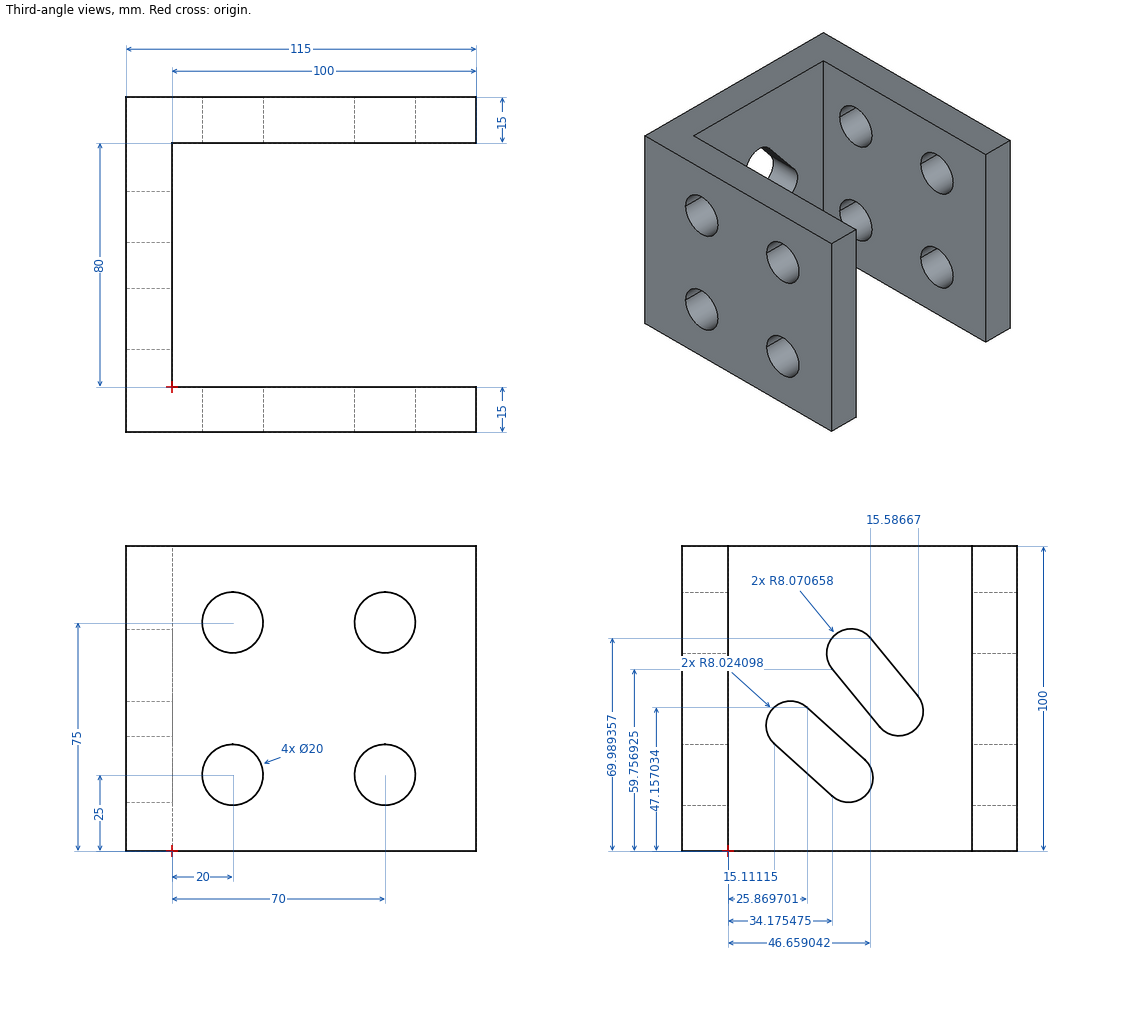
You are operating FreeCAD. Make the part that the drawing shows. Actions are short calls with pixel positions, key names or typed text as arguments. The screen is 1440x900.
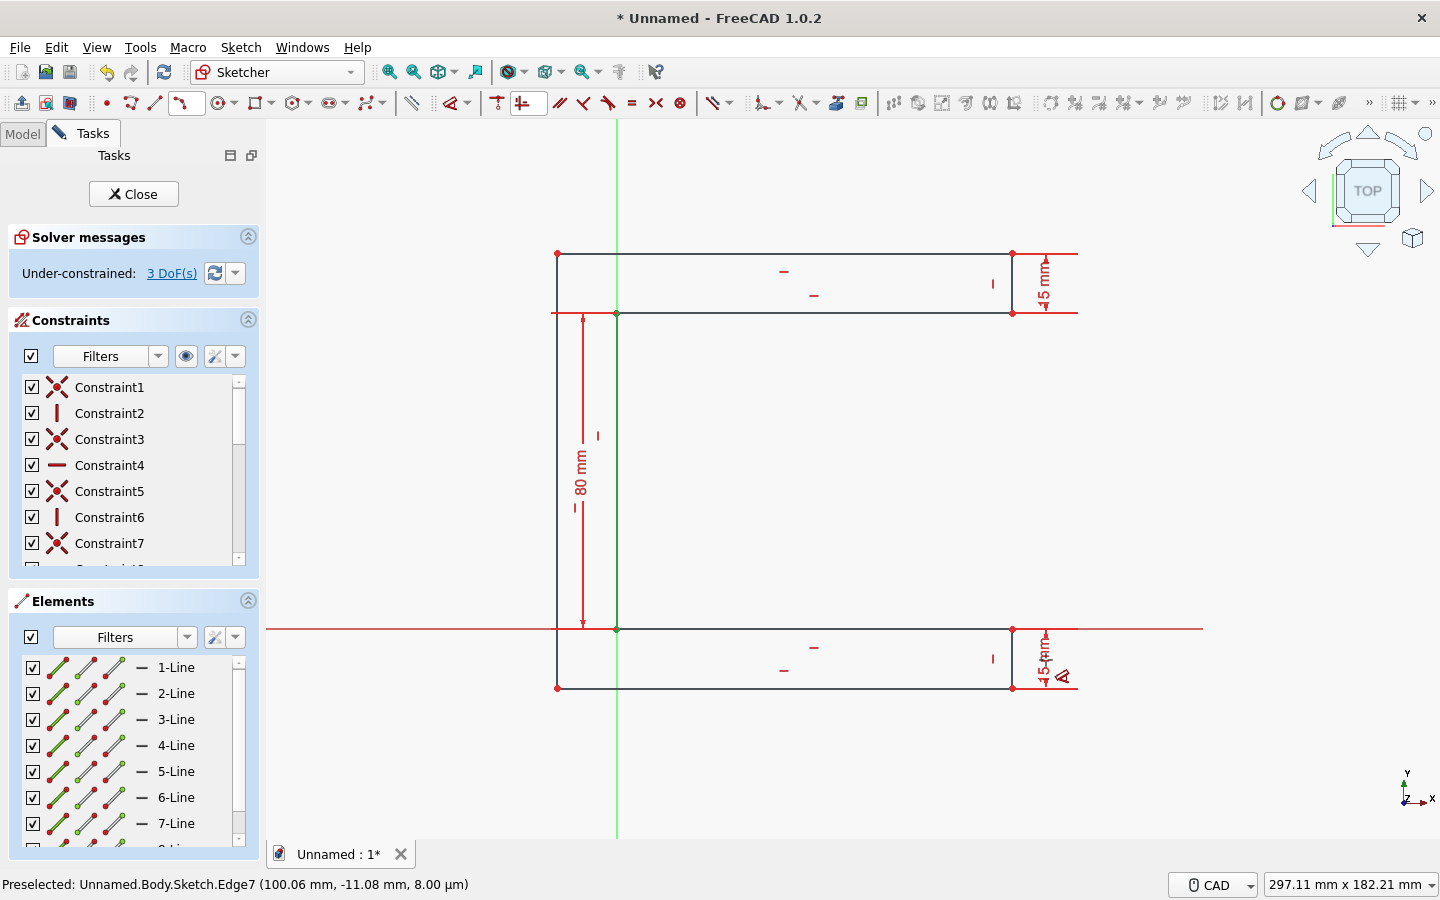
click(735, 313)
click(814, 279)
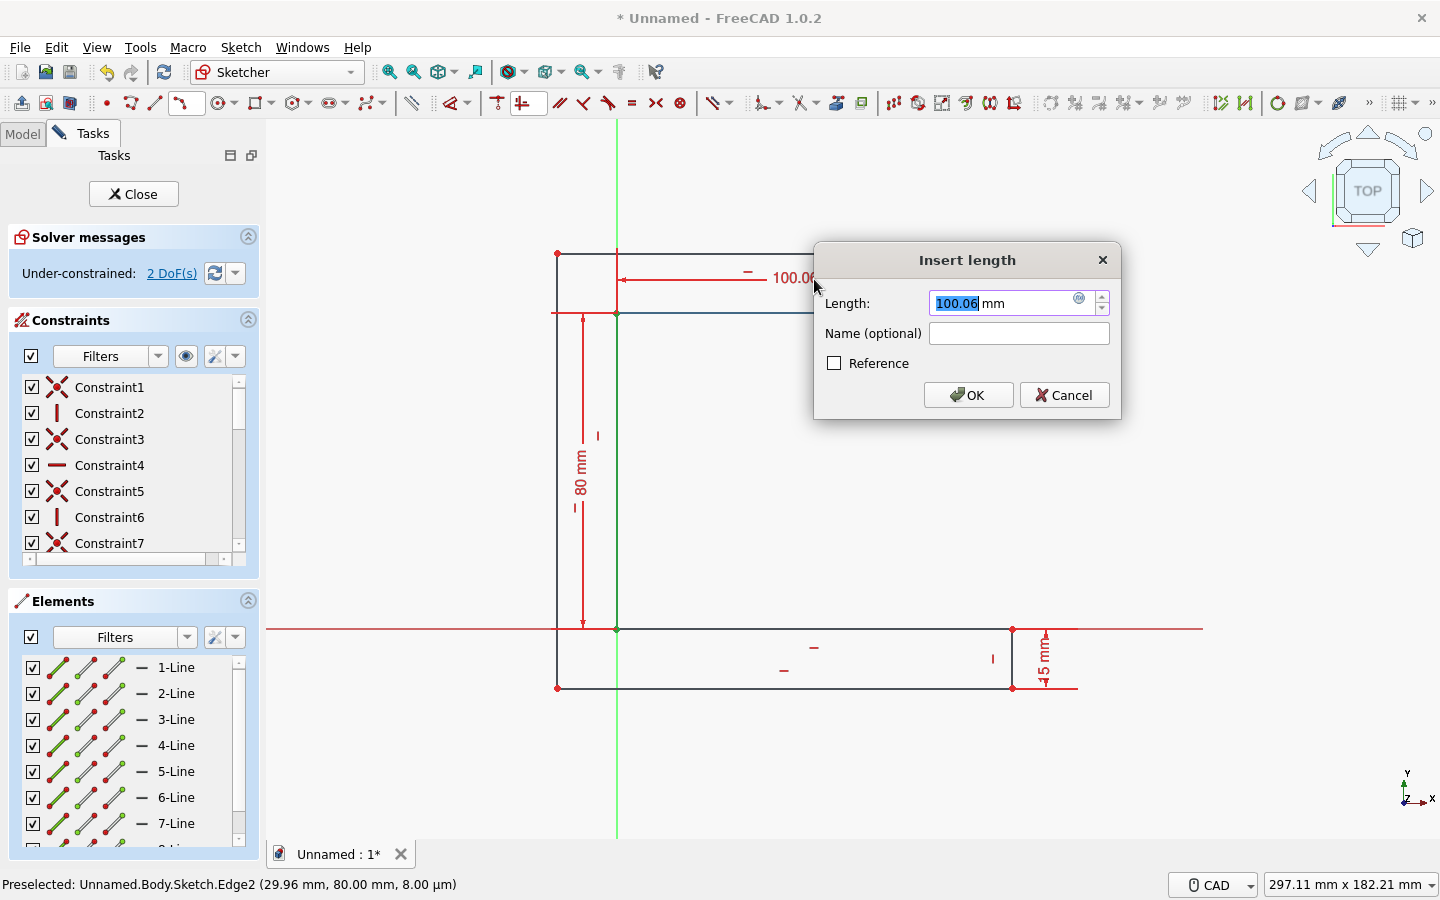
text(100)
key(Return)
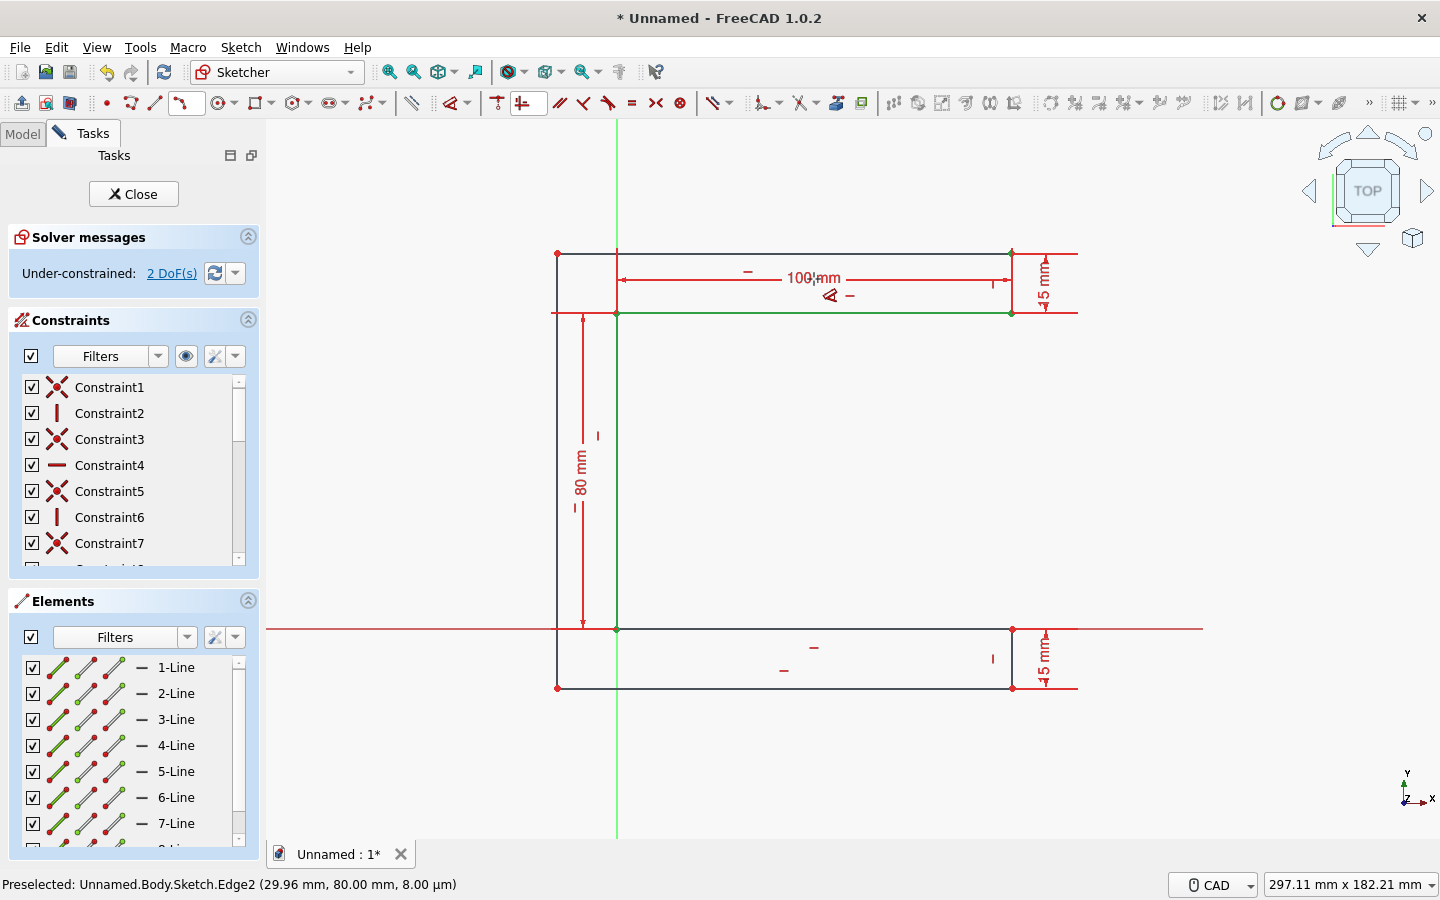
click(875, 254)
click(784, 220)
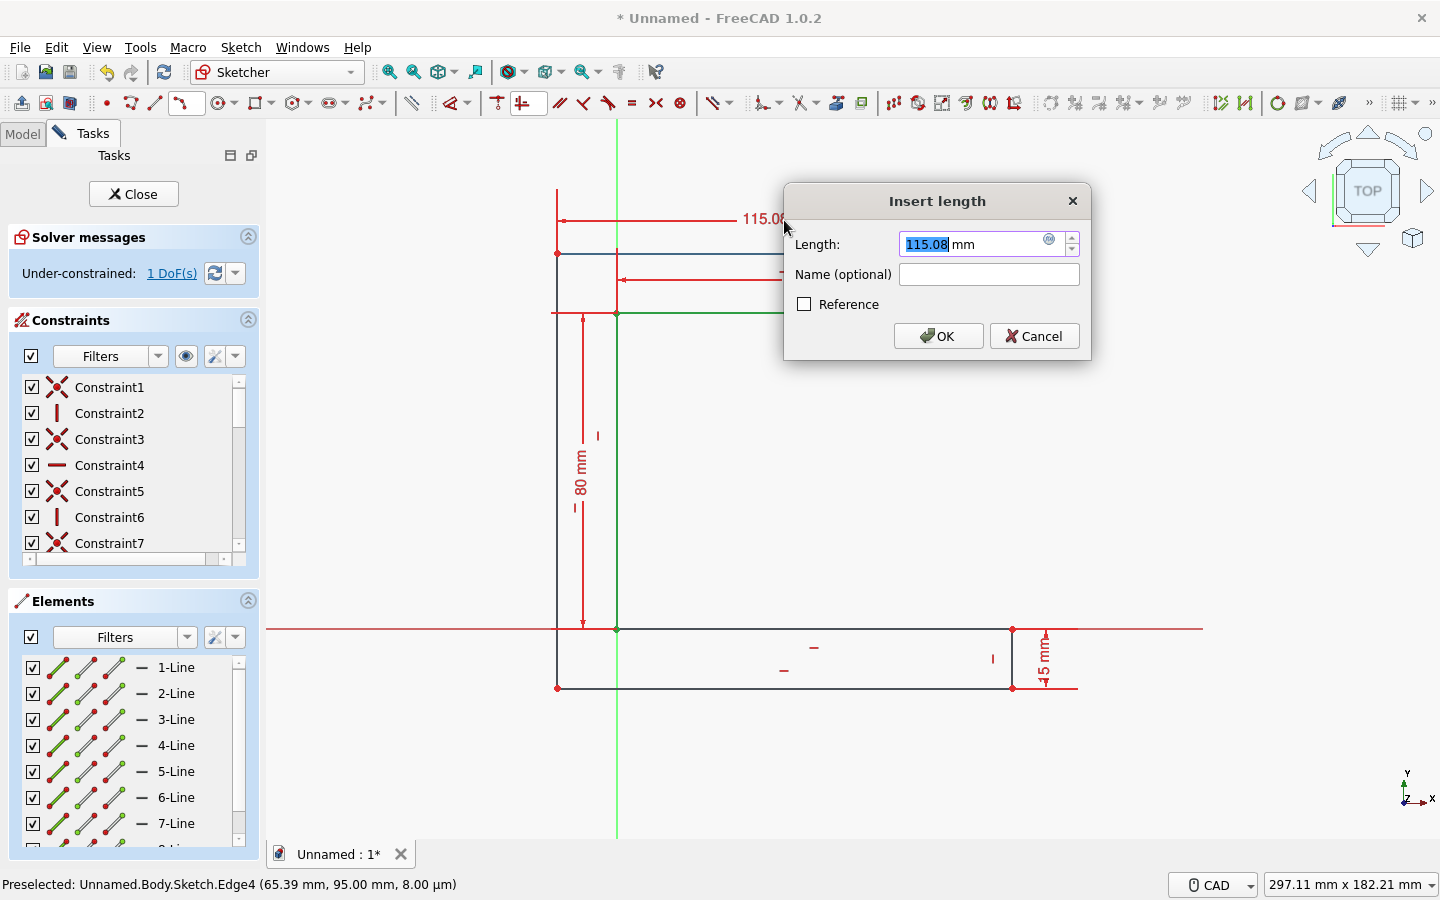
text(115)
key(Return)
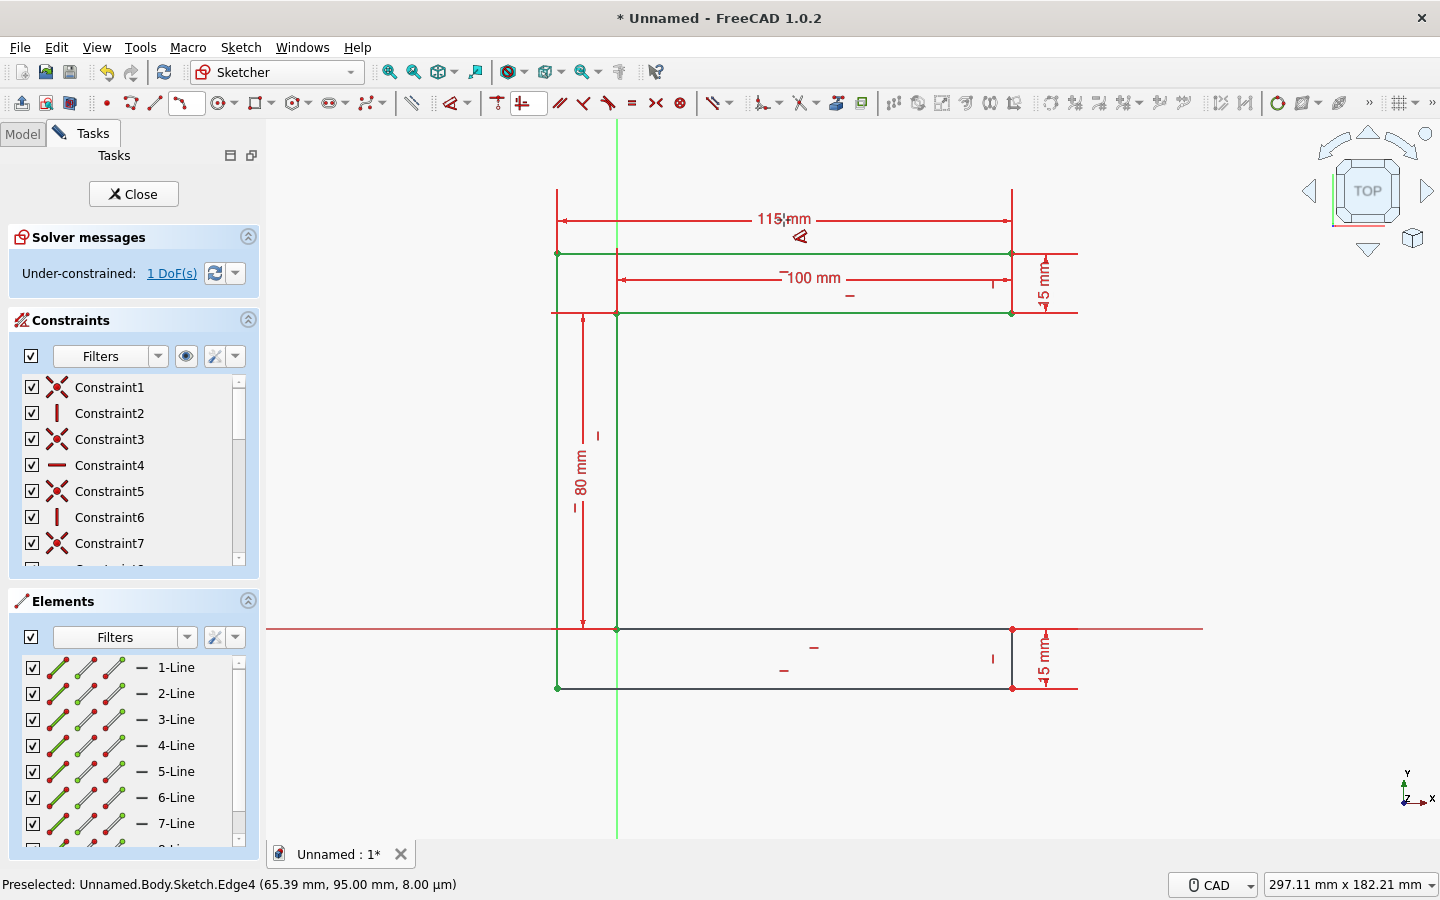
click(694, 689)
click(785, 723)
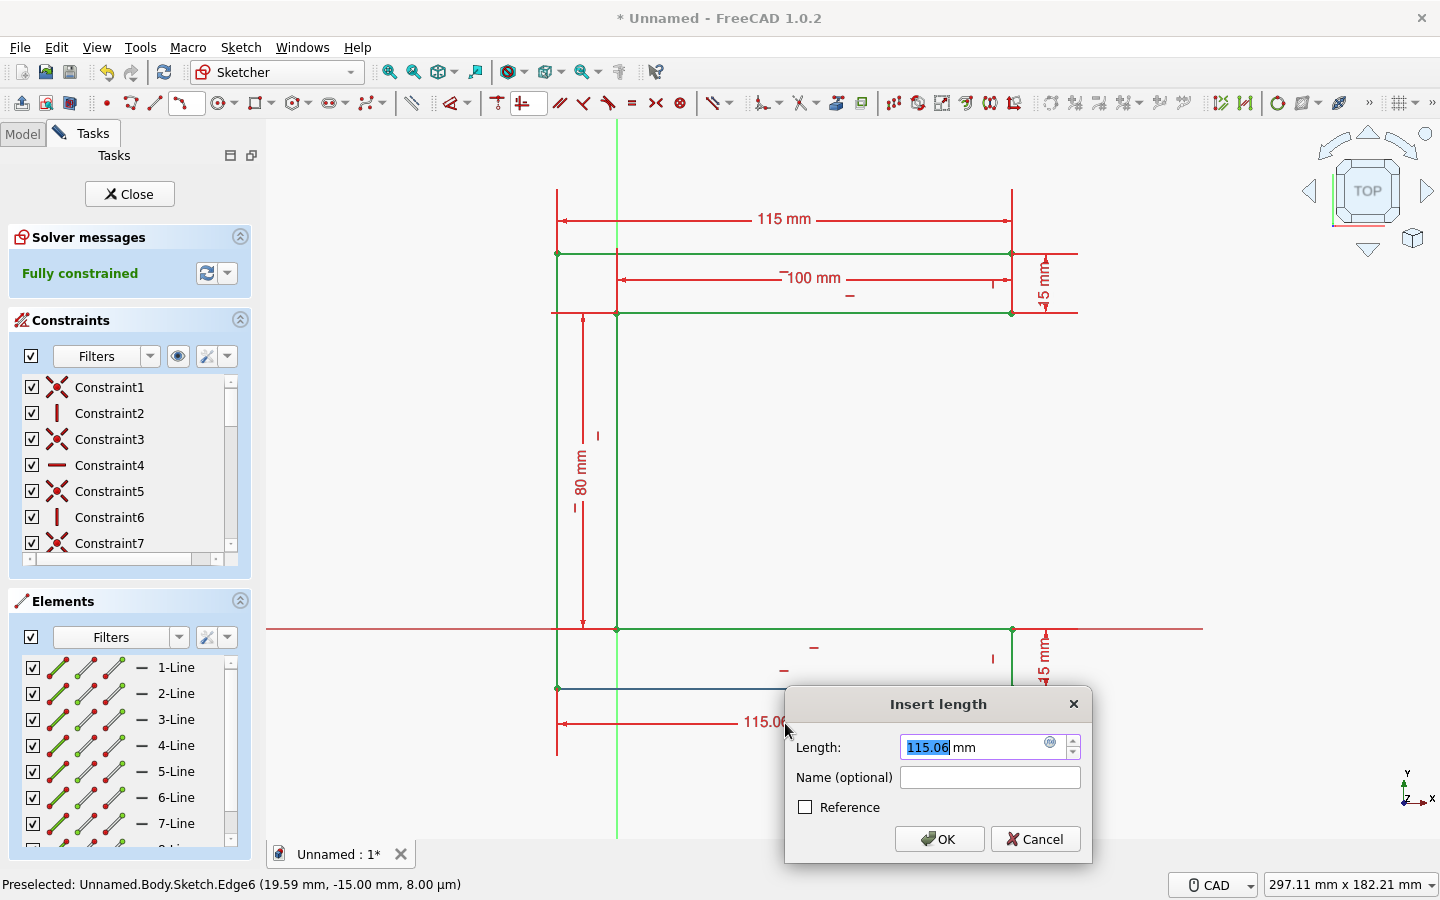
text(115)
key(Return)
key(Escape)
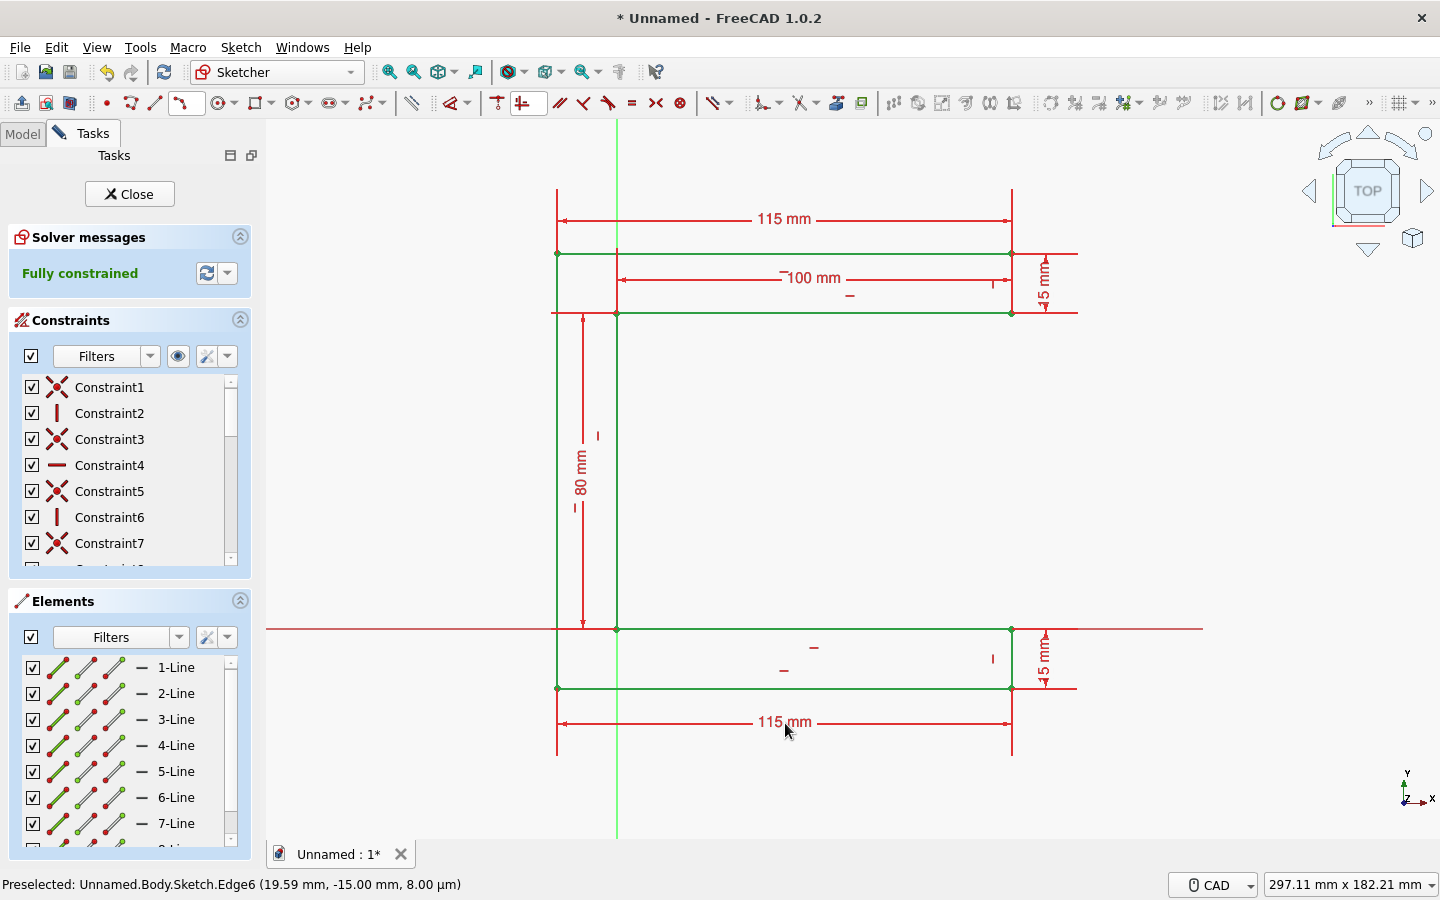
click(130, 194)